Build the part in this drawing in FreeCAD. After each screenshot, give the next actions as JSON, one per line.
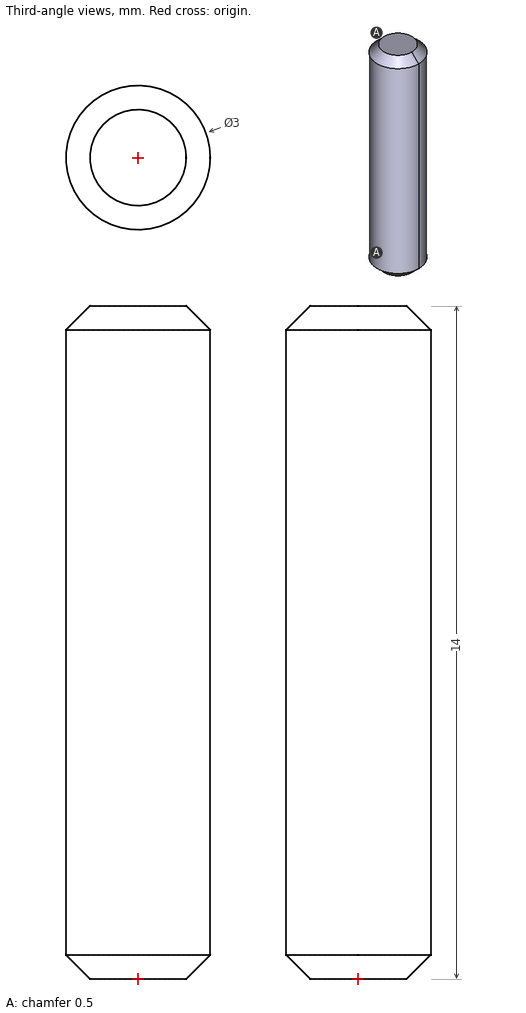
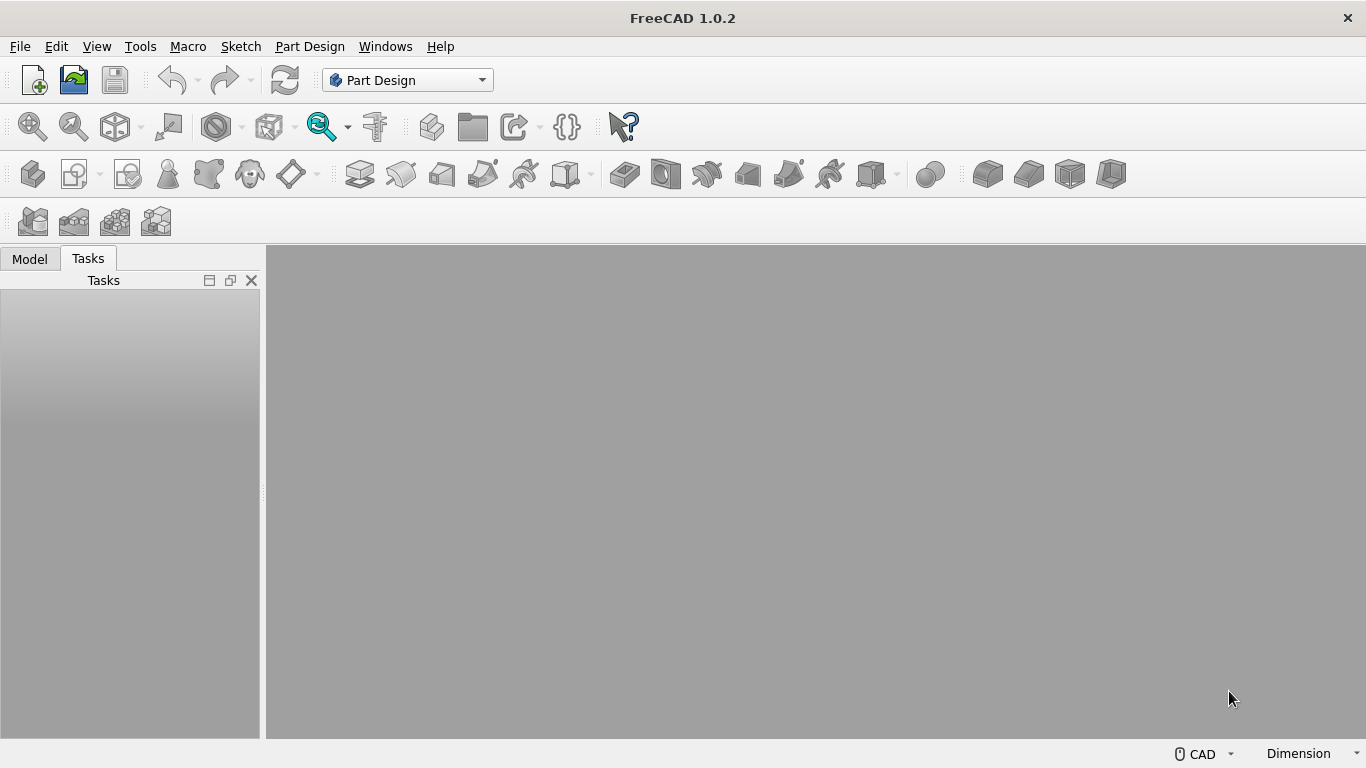
{"action": "key", "text": "ctrl+n"}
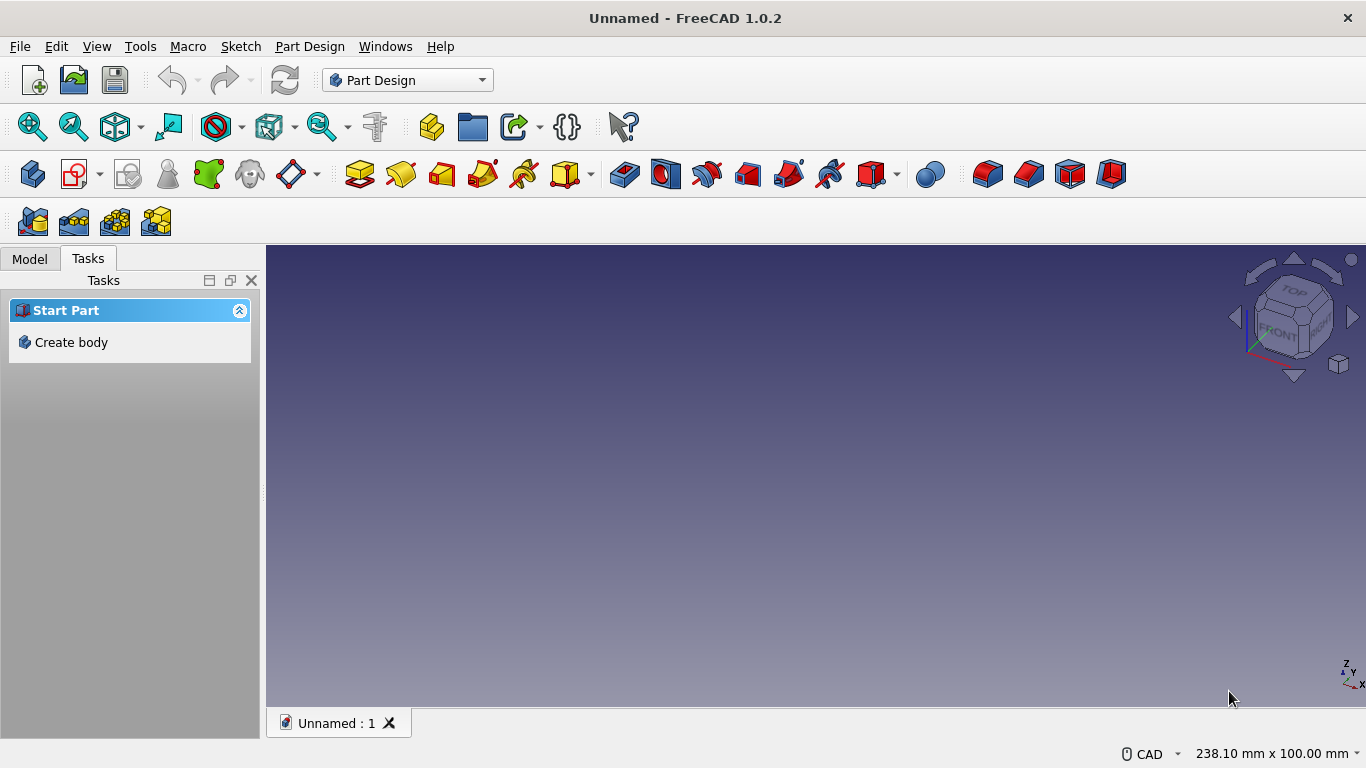
{"action": "left_click", "coordinate": [74, 174]}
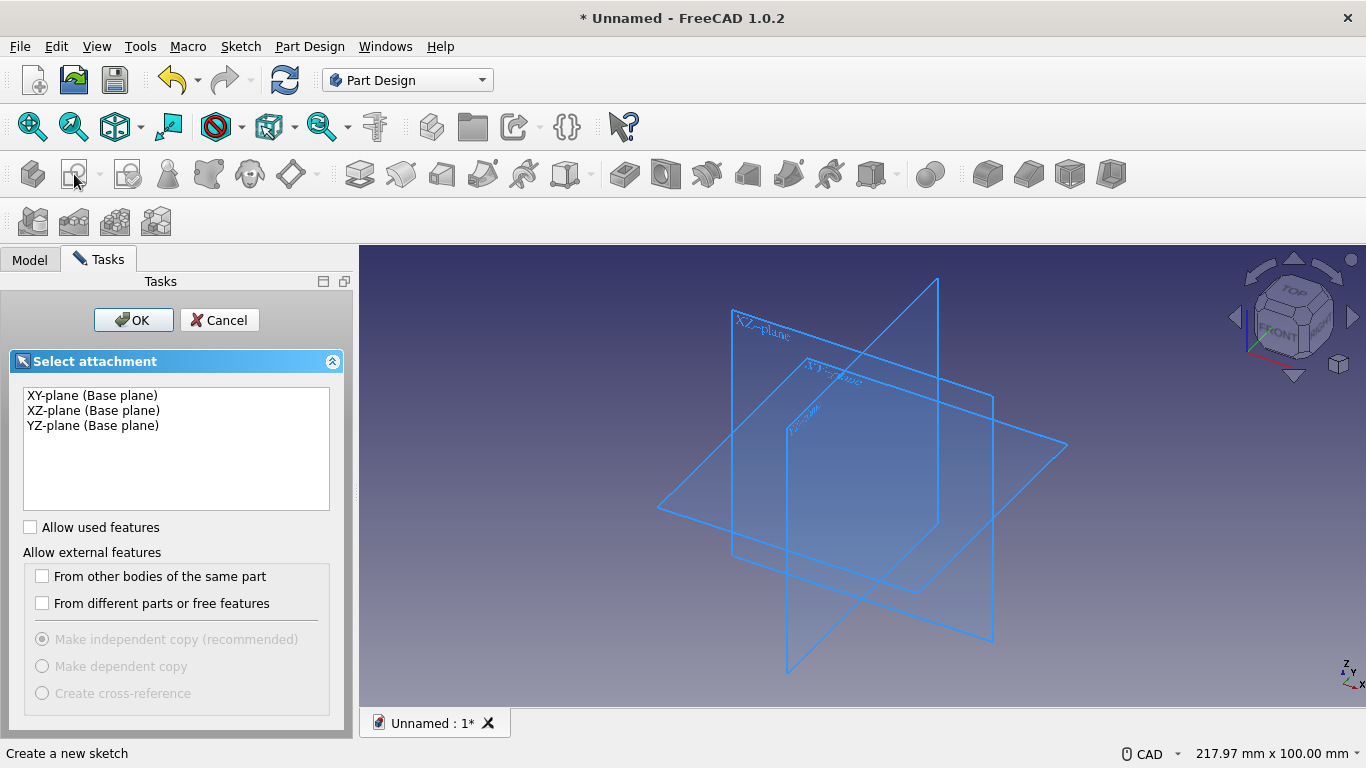
{"action": "left_click", "coordinate": [84, 396]}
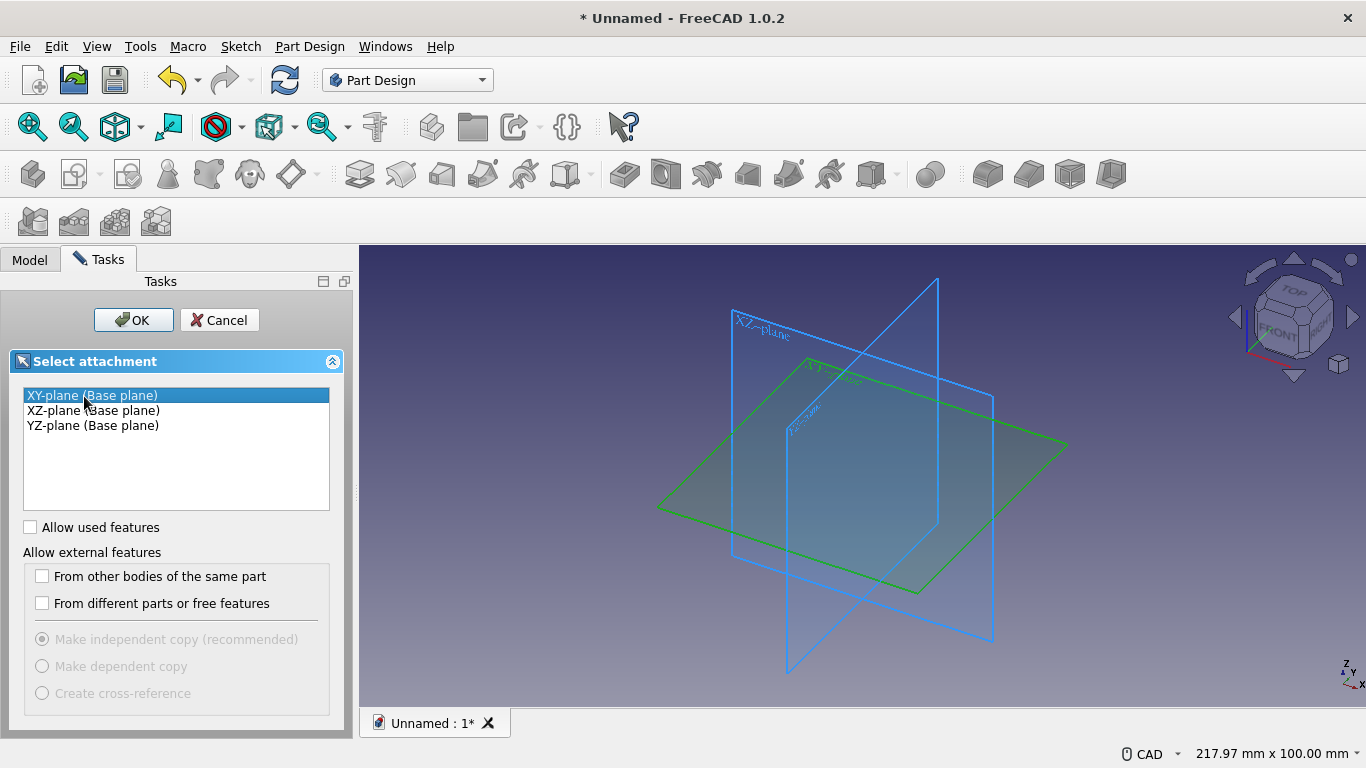
{"action": "left_click", "coordinate": [134, 320]}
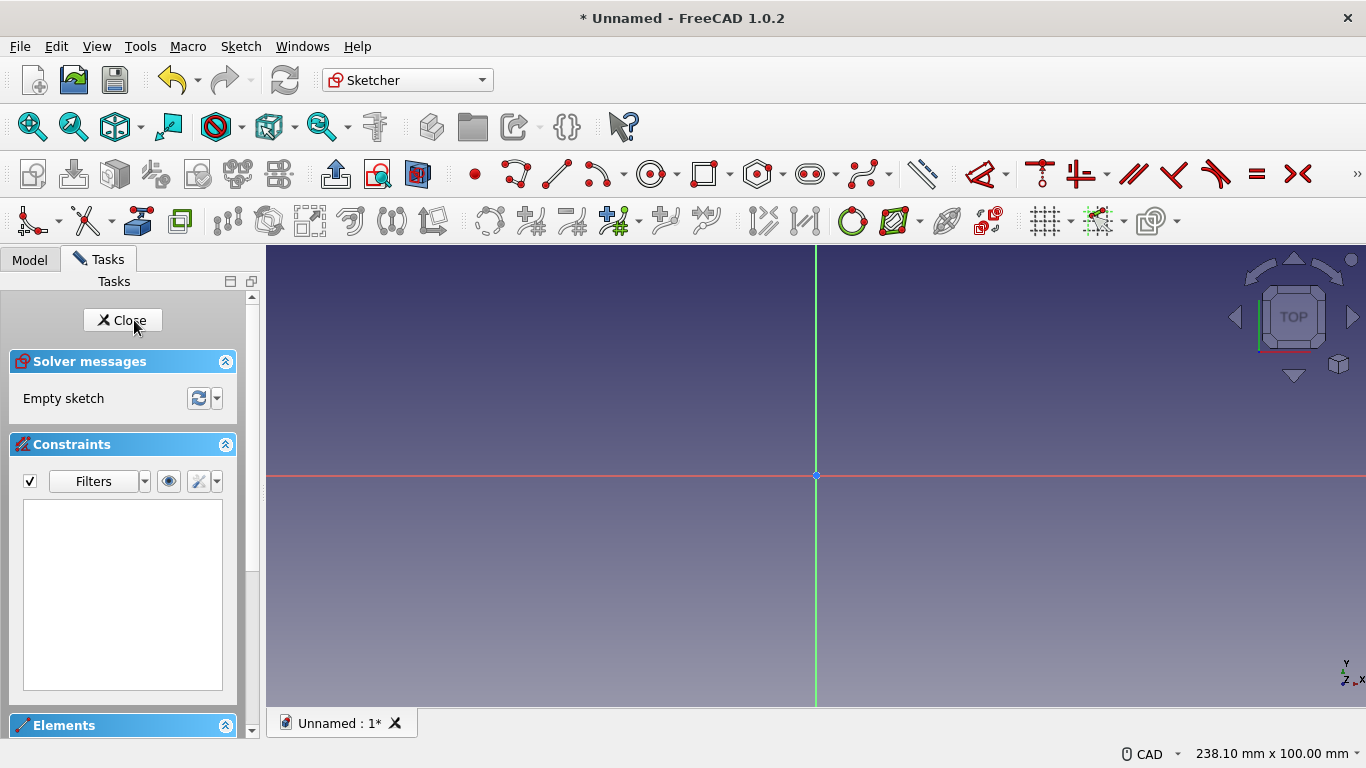
{"action": "scroll", "coordinate": [820, 476], "scroll_direction": "up", "scroll_amount": 15}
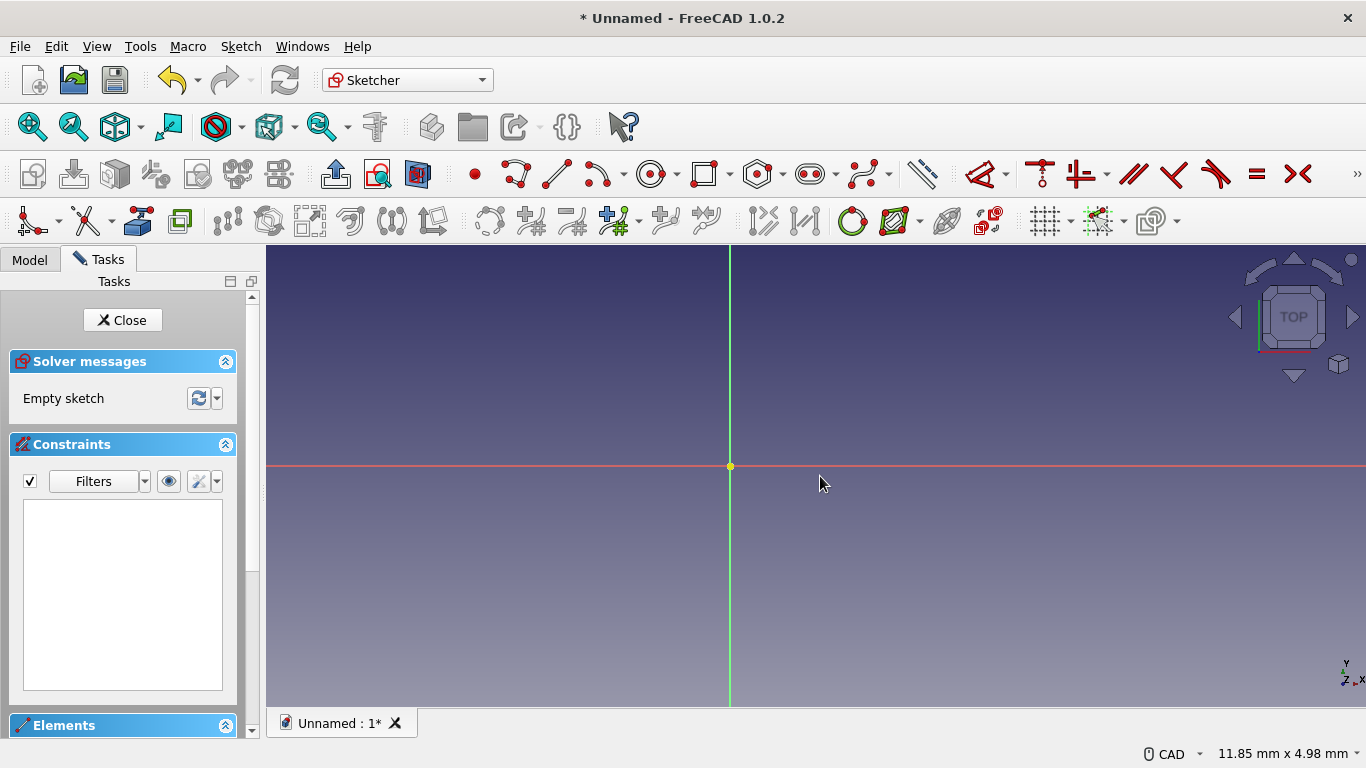
{"action": "left_click", "coordinate": [650, 174]}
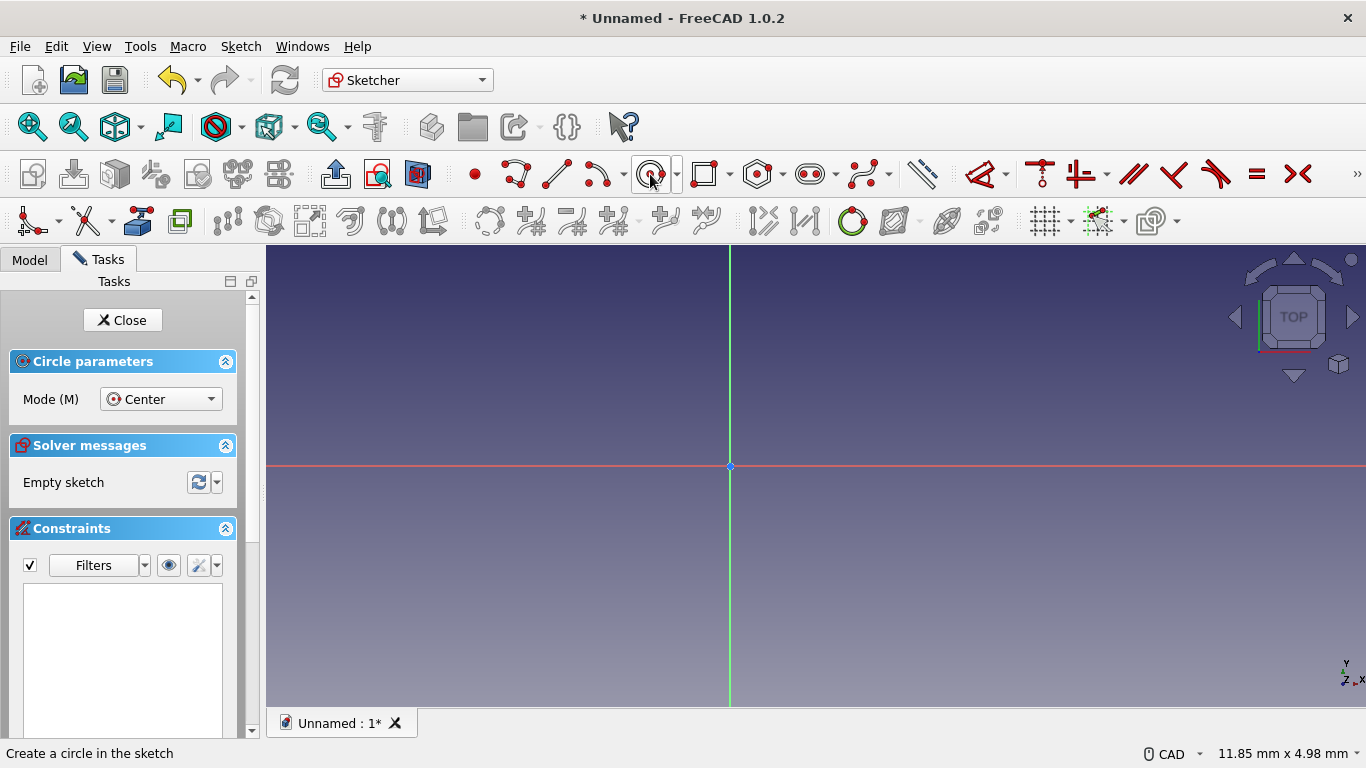
{"action": "left_click", "coordinate": [730, 466]}
{"action": "mouse_move", "coordinate": [828, 368]}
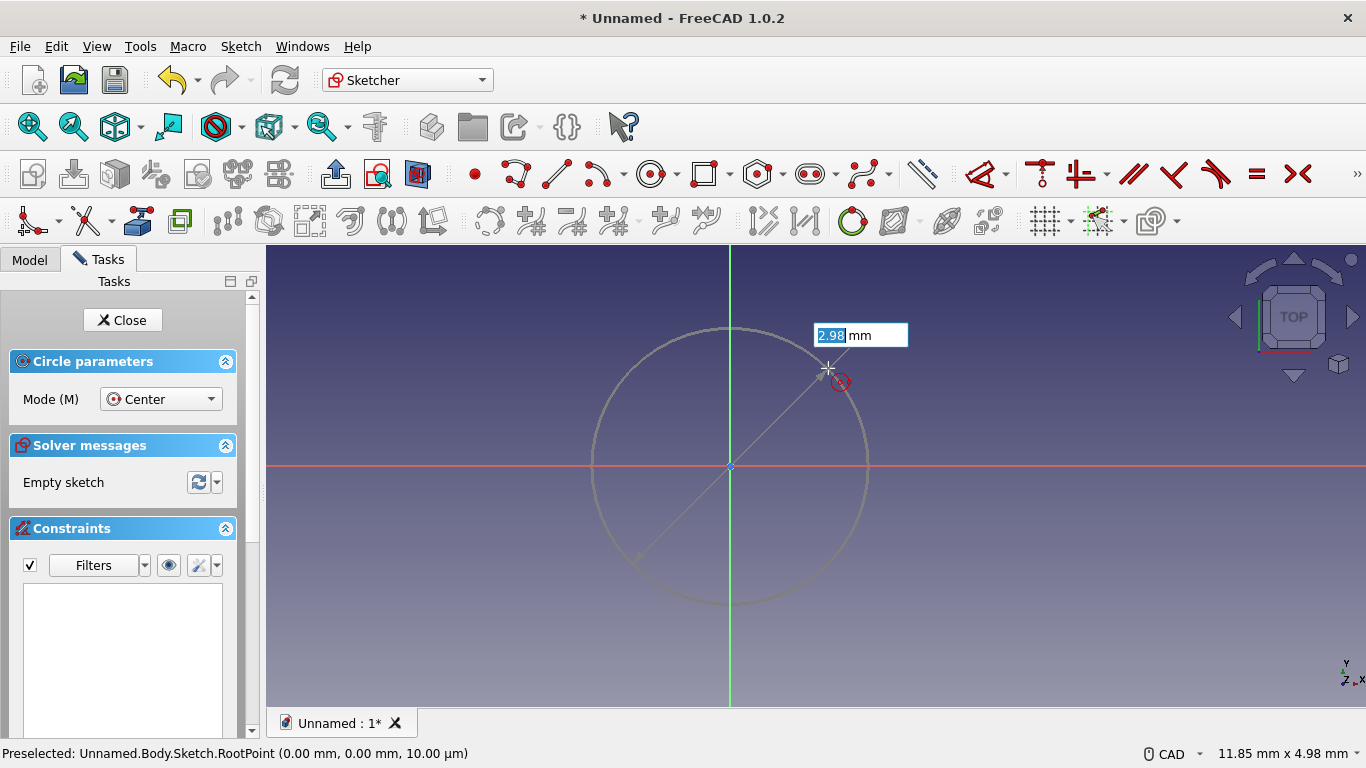
{"action": "type", "text": "3"}
{"action": "key", "text": "Return"}
{"action": "key", "text": "Escape"}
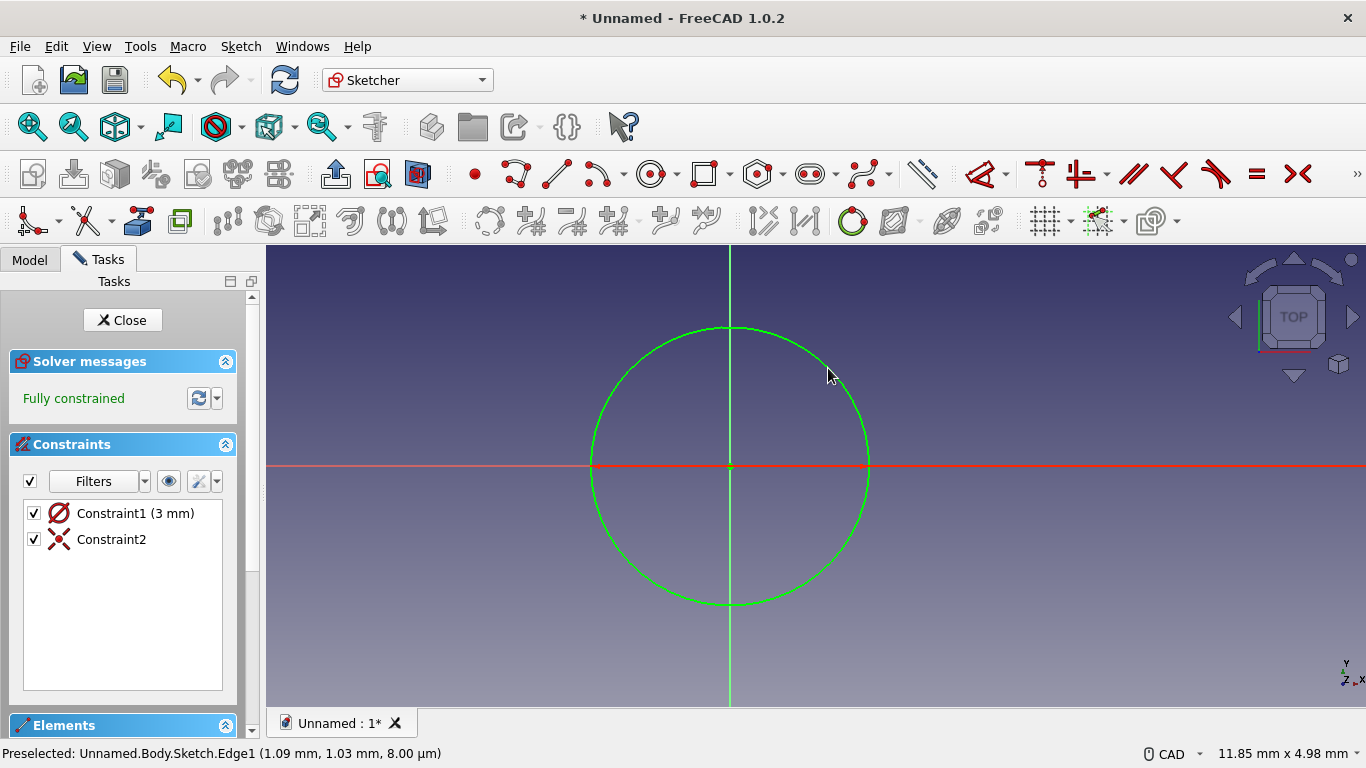
{"action": "left_click", "coordinate": [123, 320]}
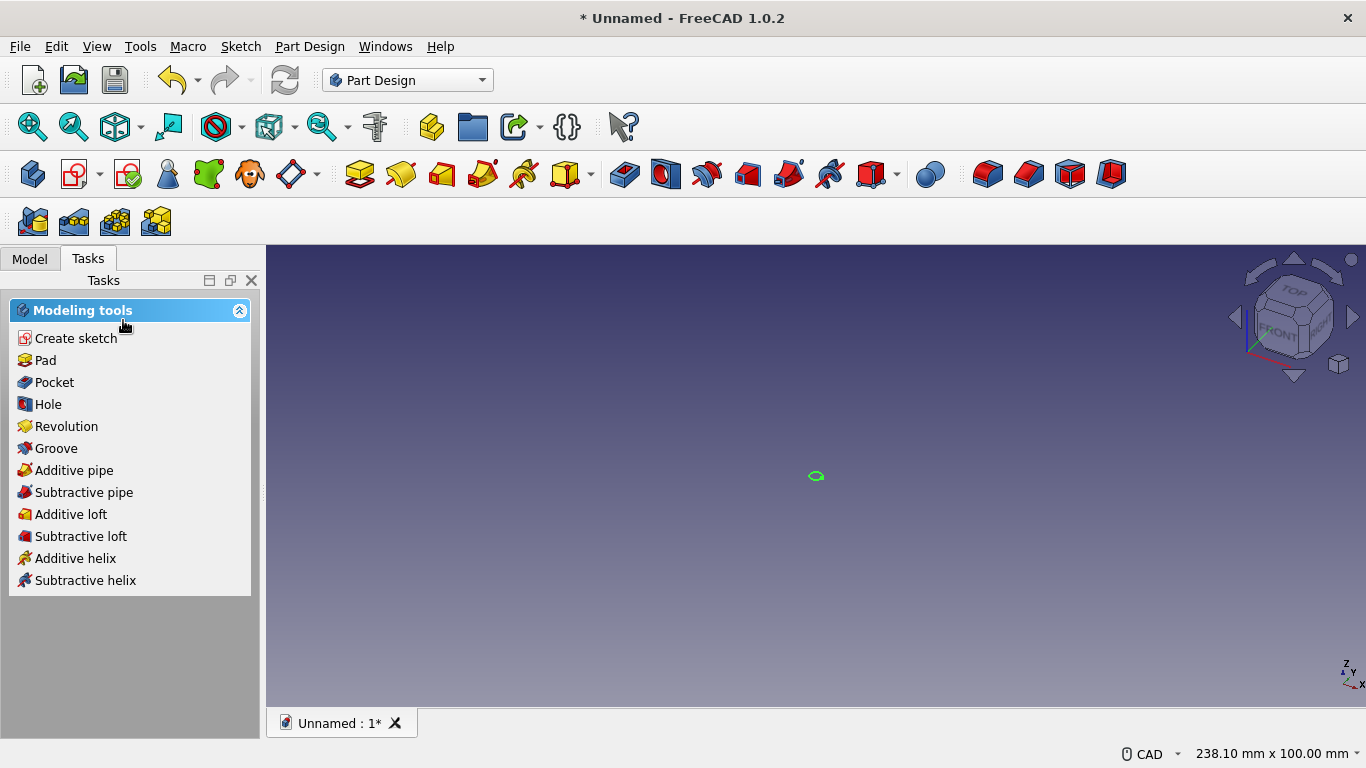
{"action": "left_click", "coordinate": [360, 174]}